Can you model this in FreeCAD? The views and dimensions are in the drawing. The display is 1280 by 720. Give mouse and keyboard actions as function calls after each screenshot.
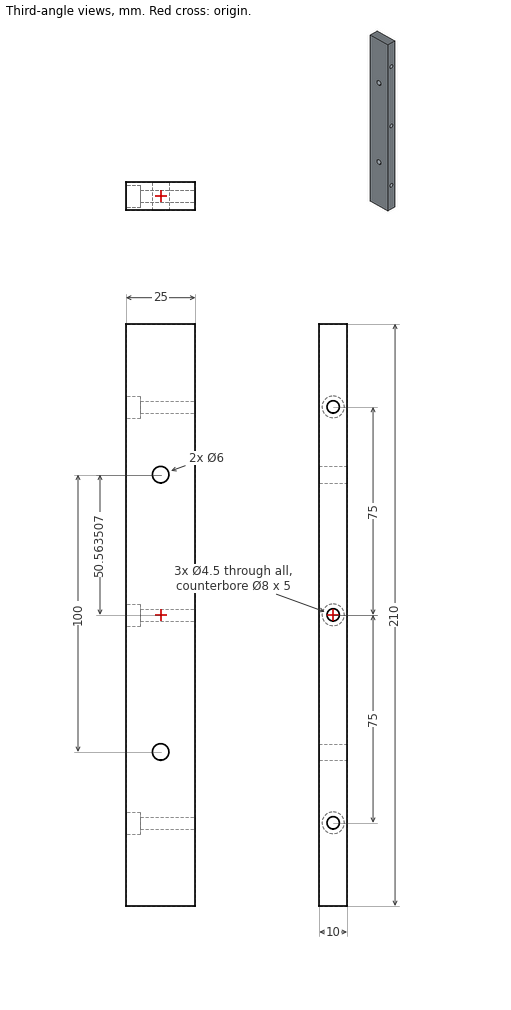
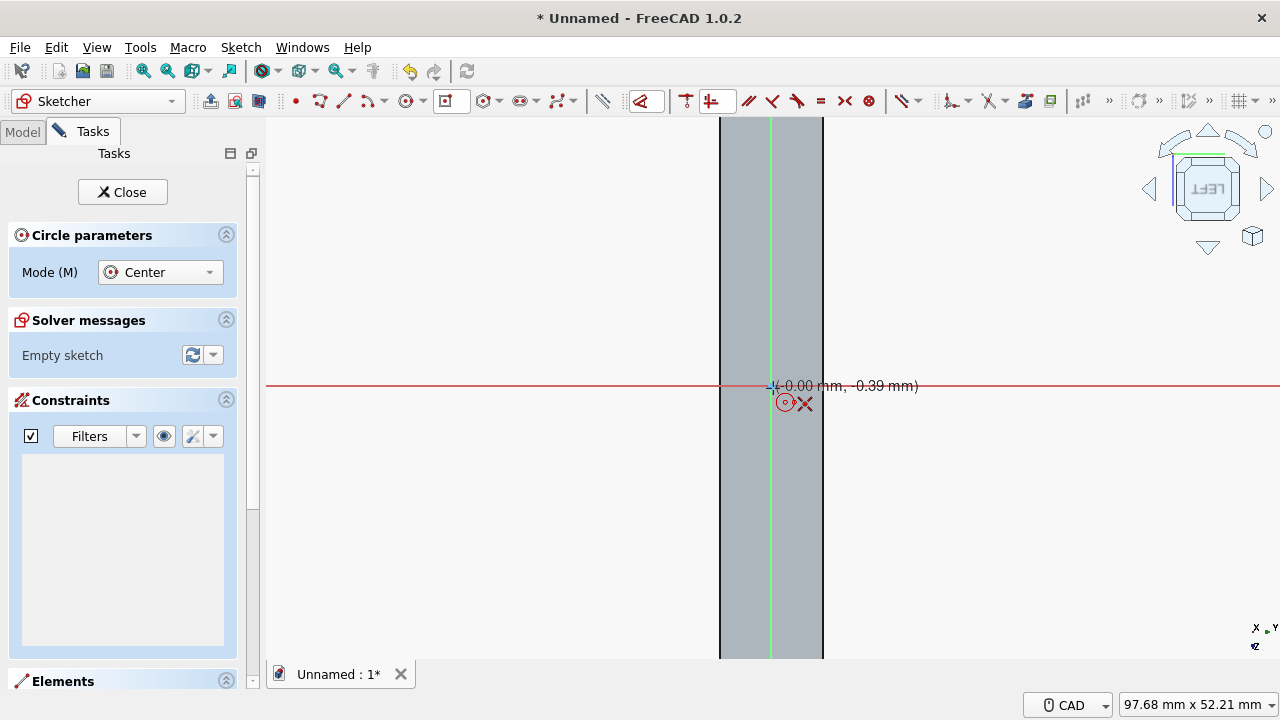
scroll(688, 388, down, 8)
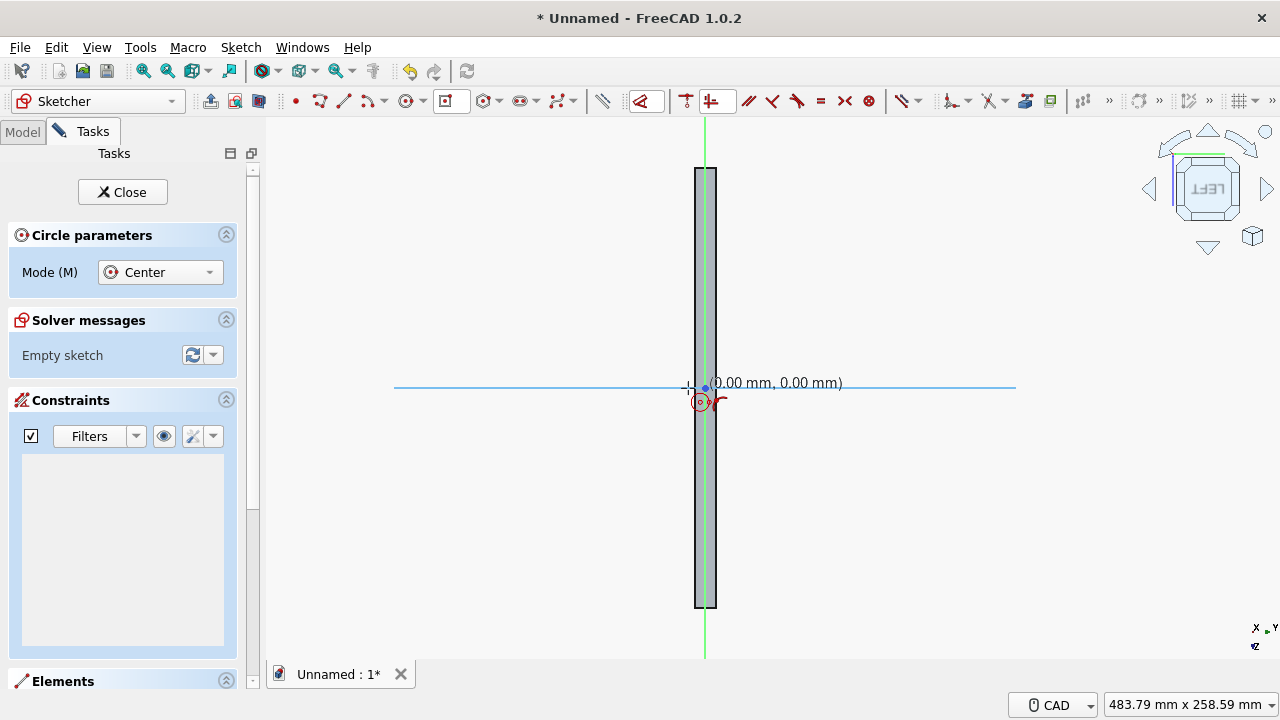
click(705, 388)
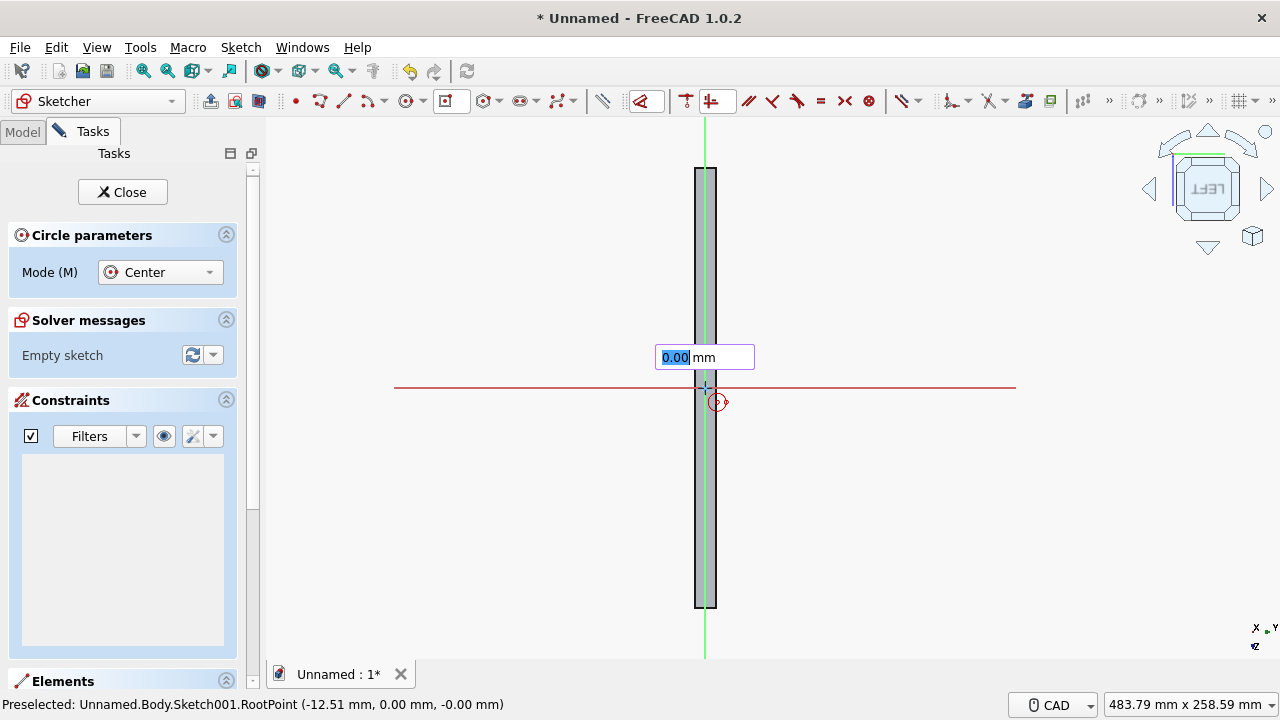
scroll(709, 385, up, 8)
move(705, 382)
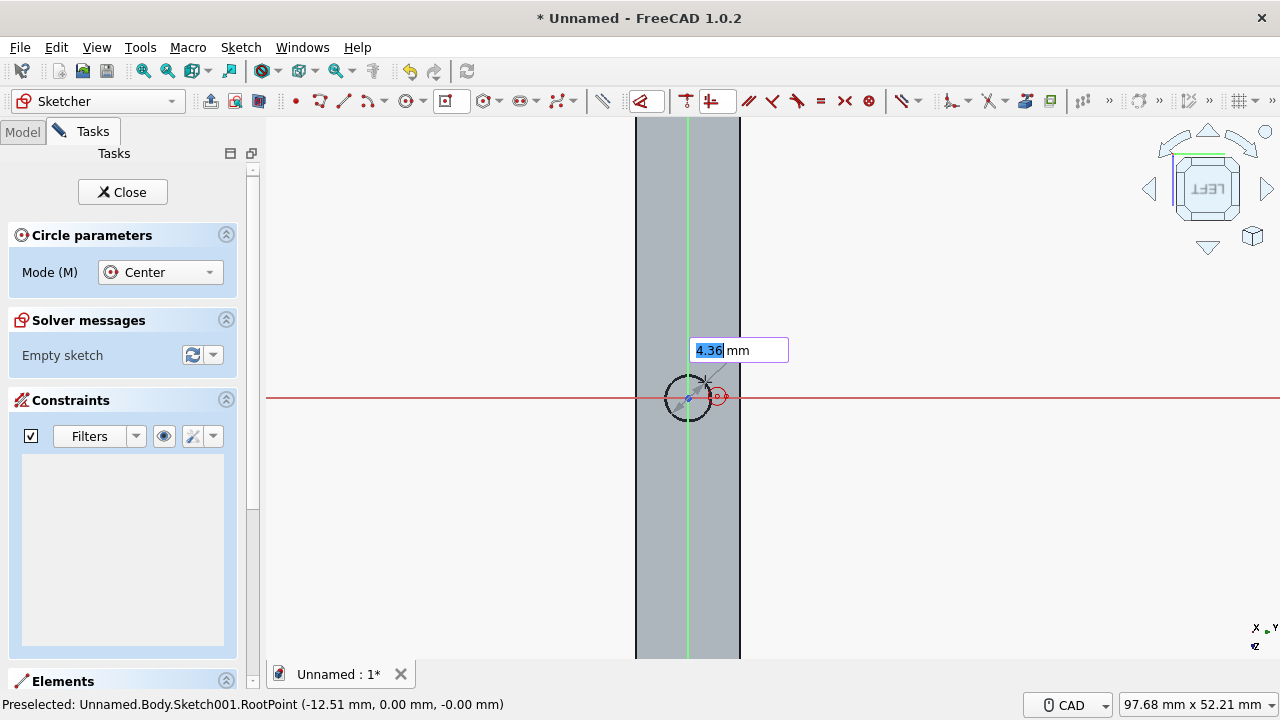
text(4.5)
key(Return)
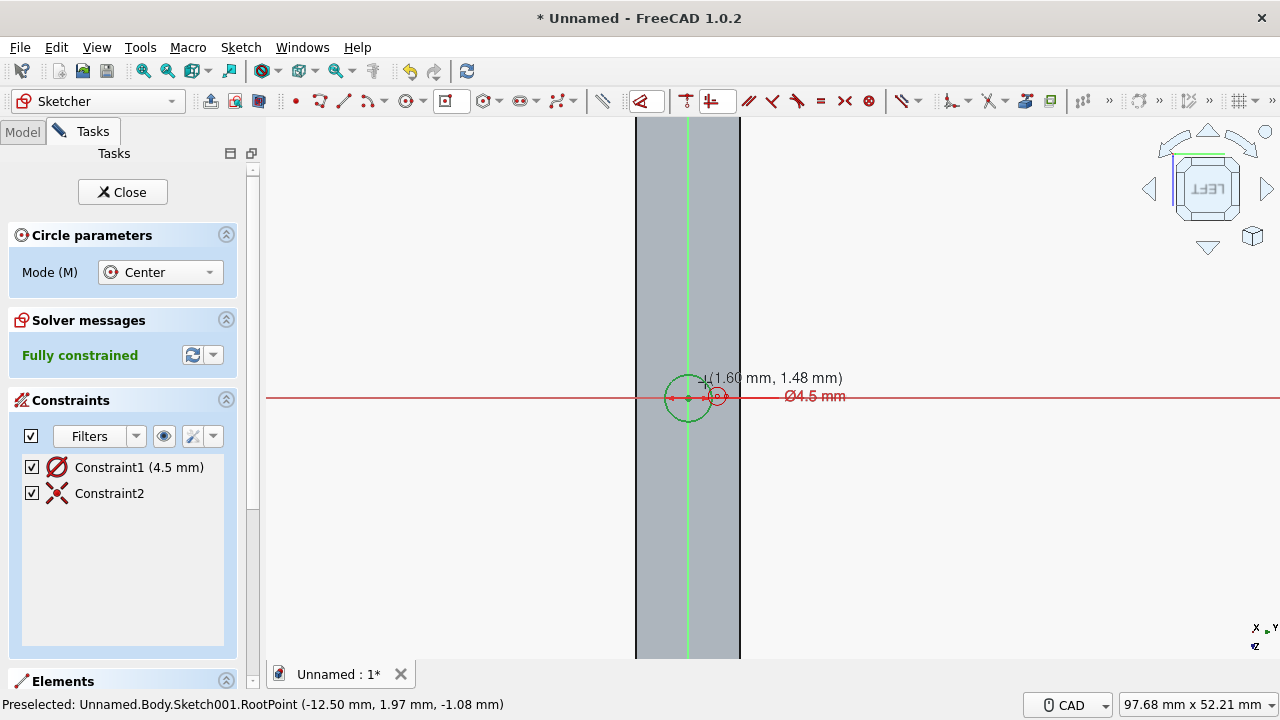
scroll(709, 385, down, 8)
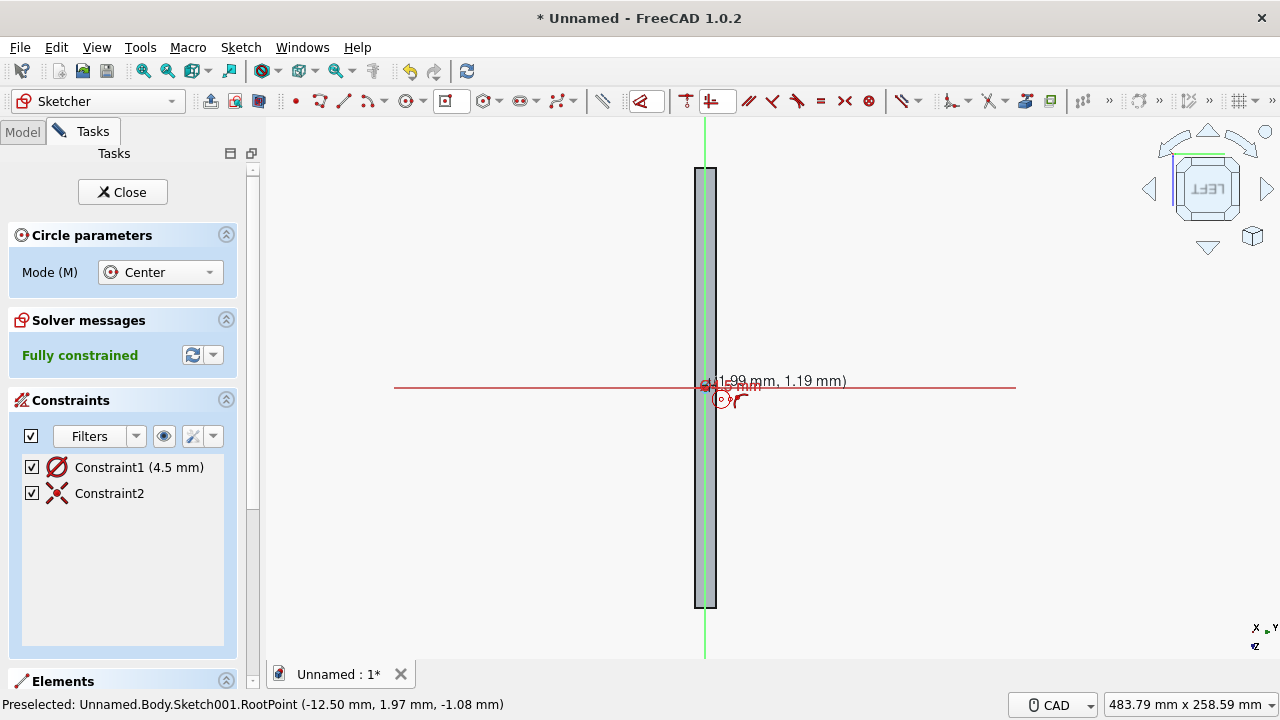
scroll(705, 231, up, 8)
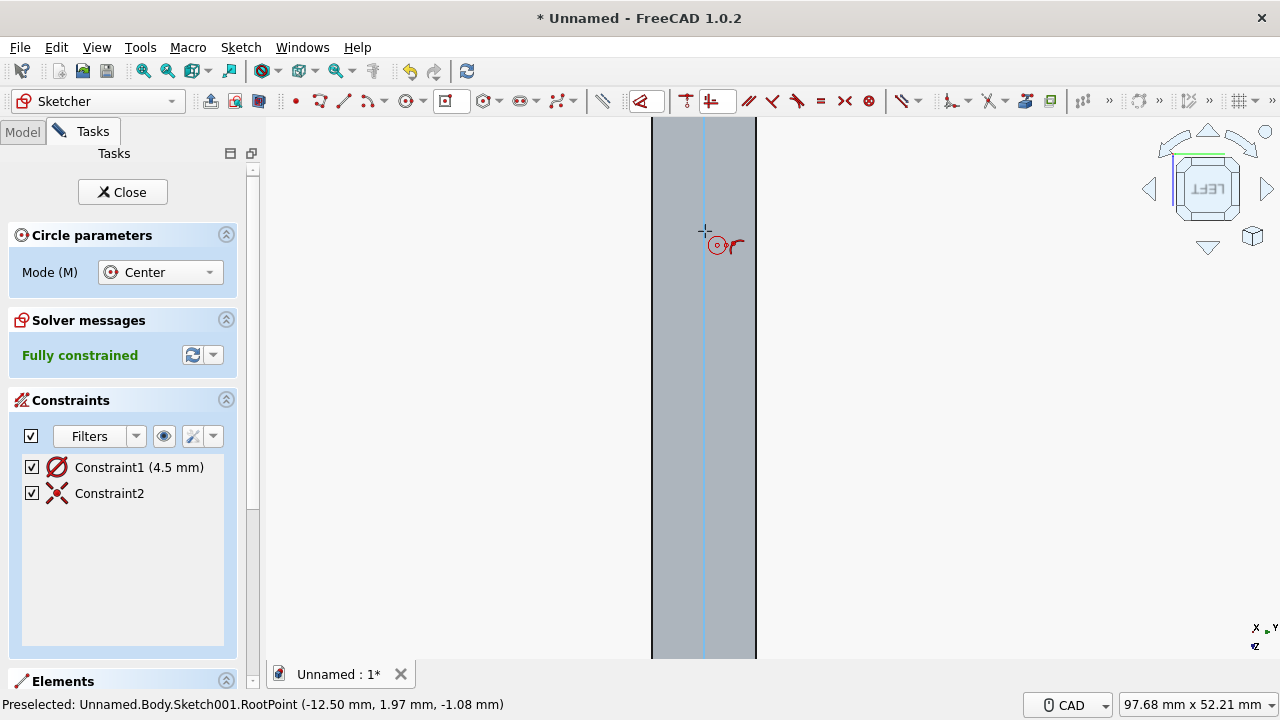
scroll(705, 231, down, 8)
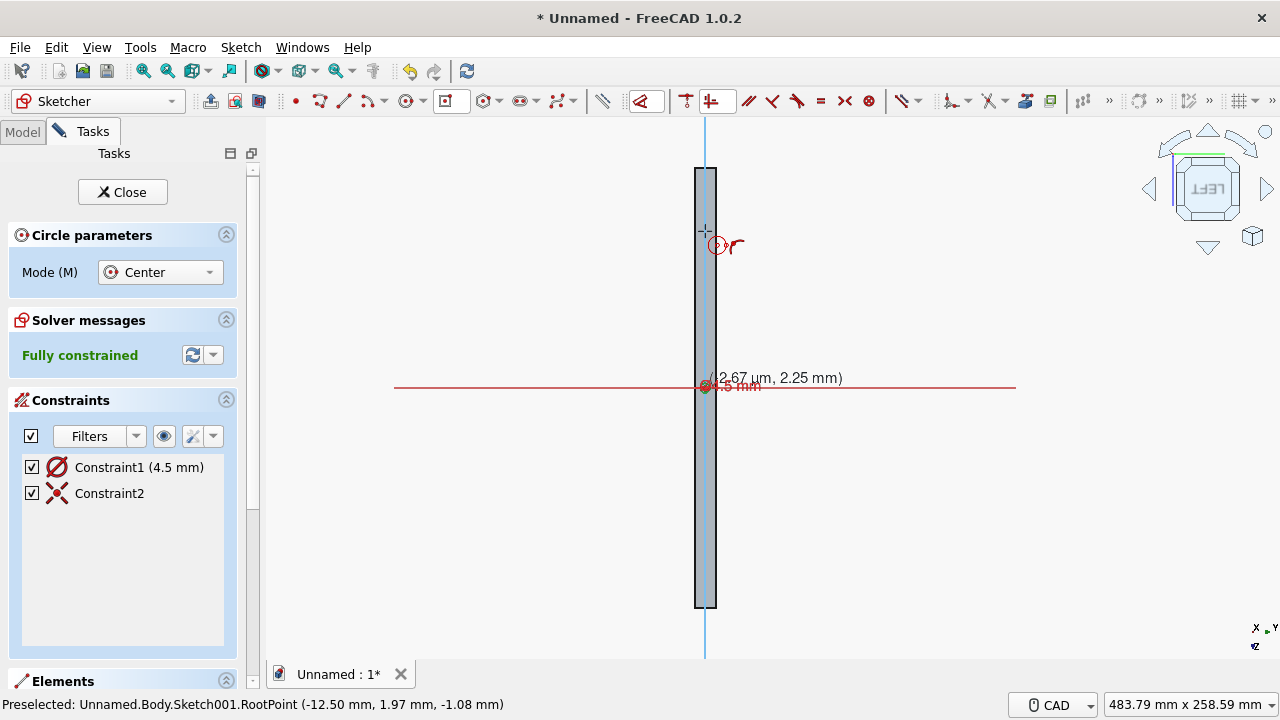
click(705, 231)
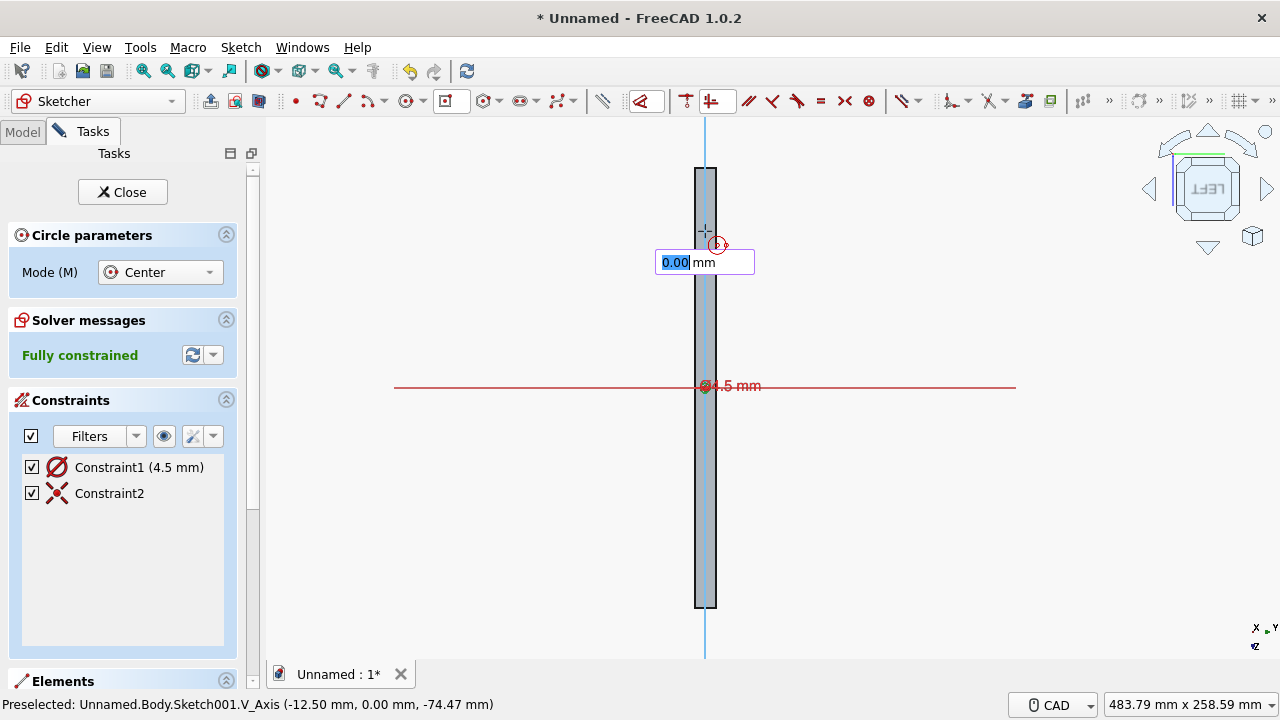
scroll(710, 229, up, 7)
move(707, 230)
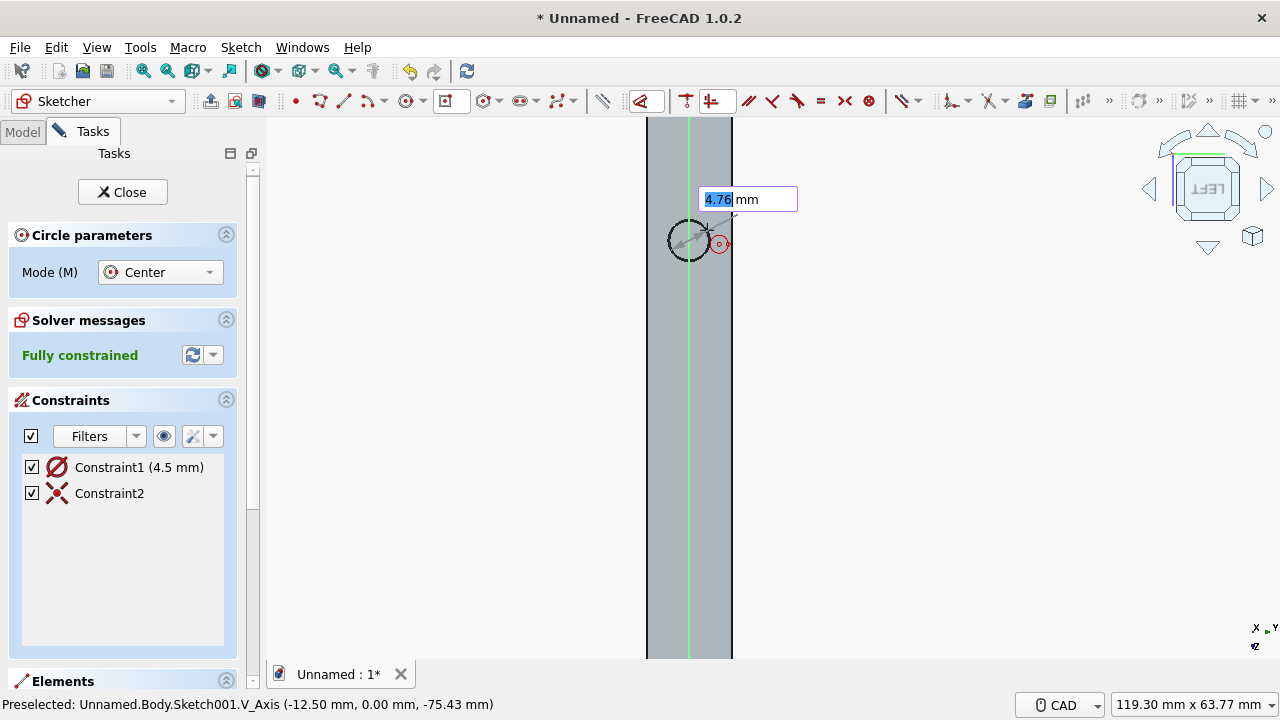
text(4.5)
key(Return)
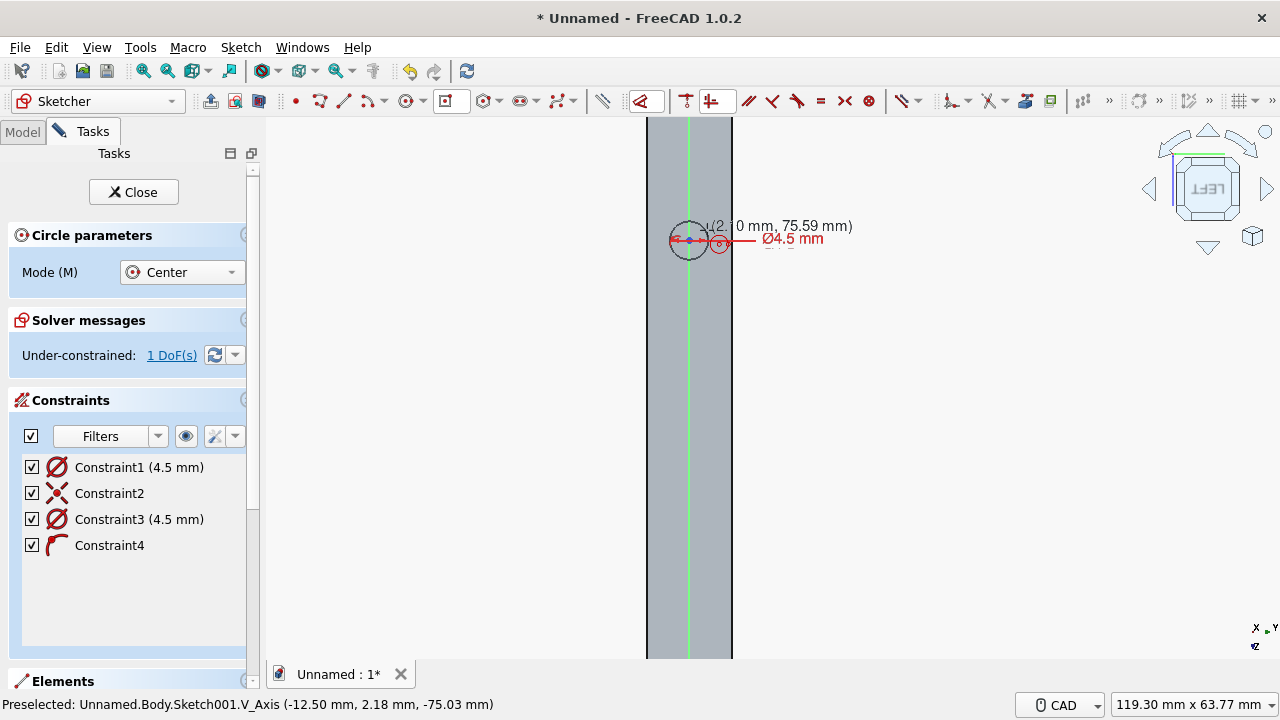
scroll(710, 229, down, 7)